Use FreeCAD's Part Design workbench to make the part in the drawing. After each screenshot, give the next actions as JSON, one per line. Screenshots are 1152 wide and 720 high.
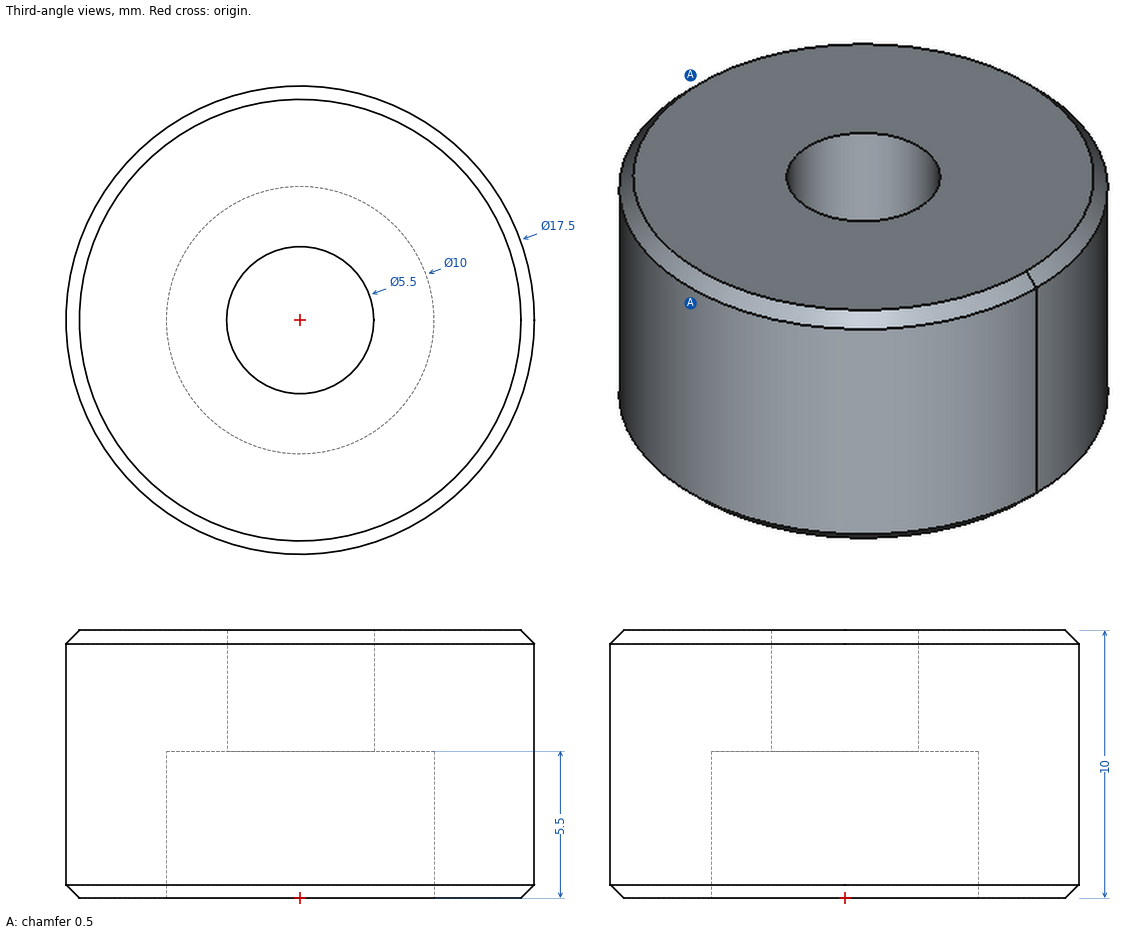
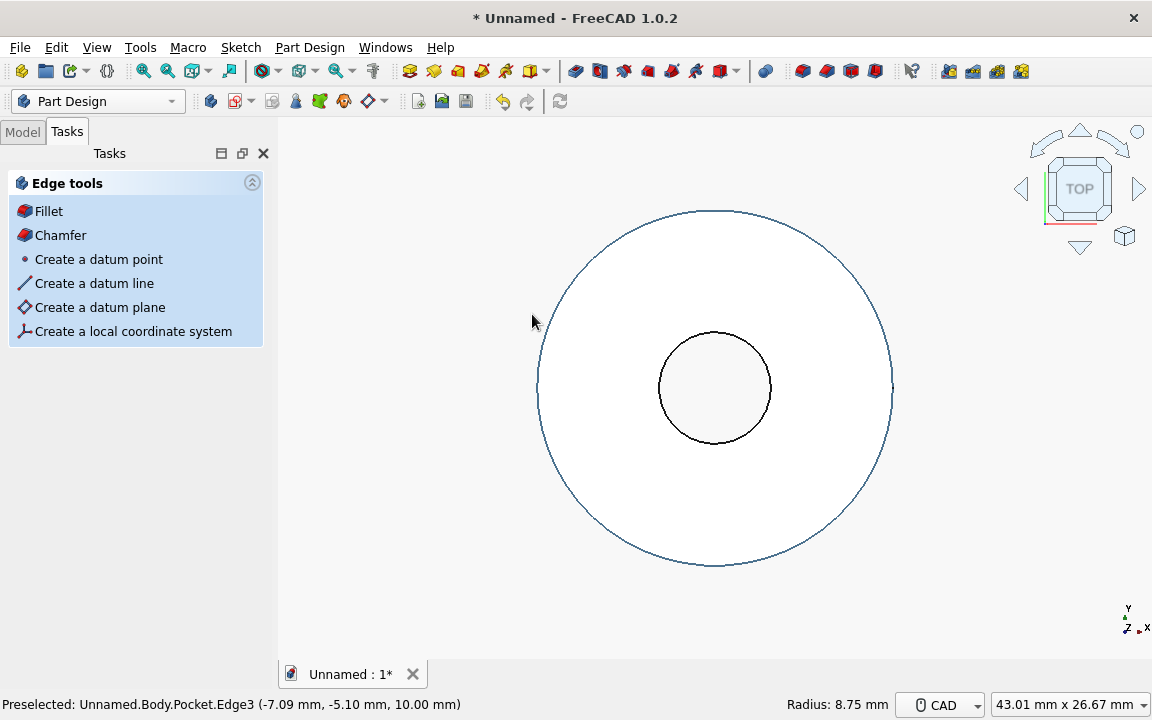
{"action": "key", "text": "1"}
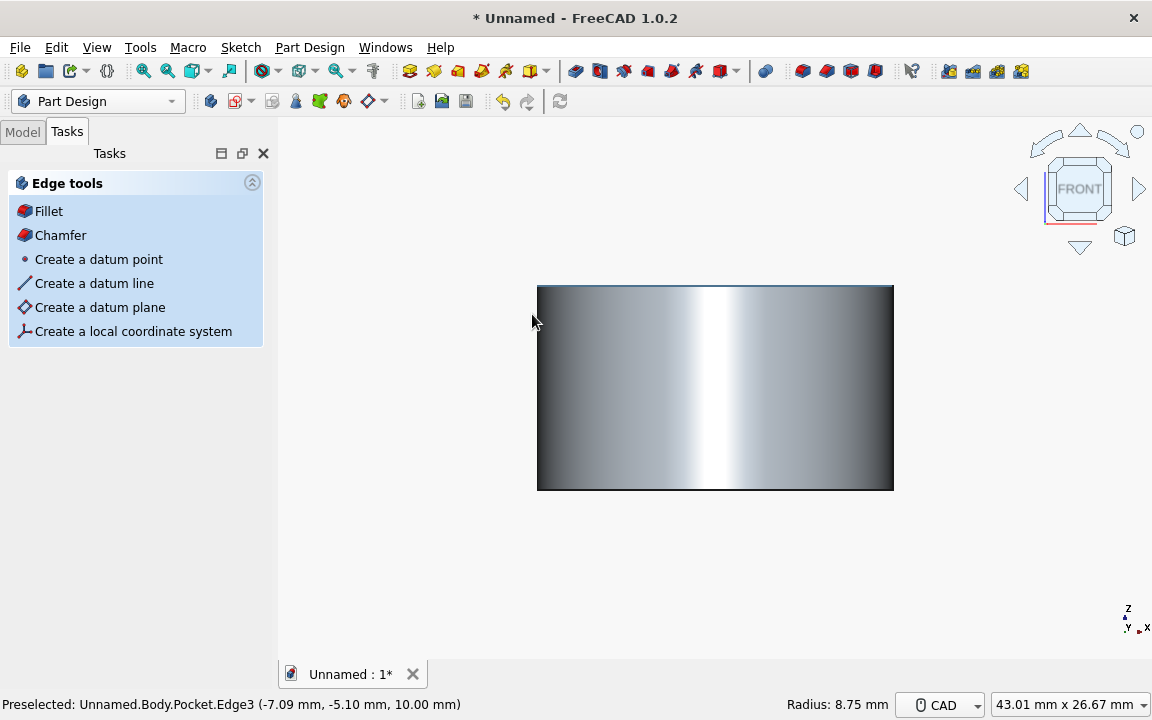
{"action": "left_click", "coordinate": [144, 72]}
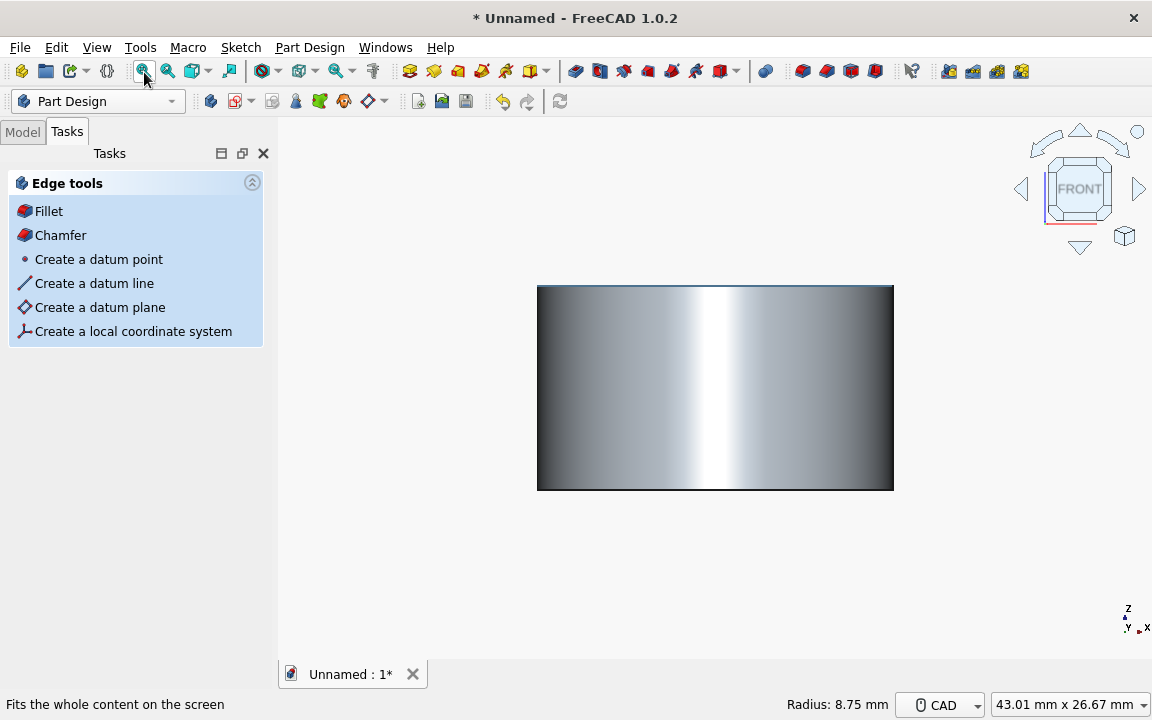
{"action": "left_click", "coordinate": [571, 489], "text": "ctrl"}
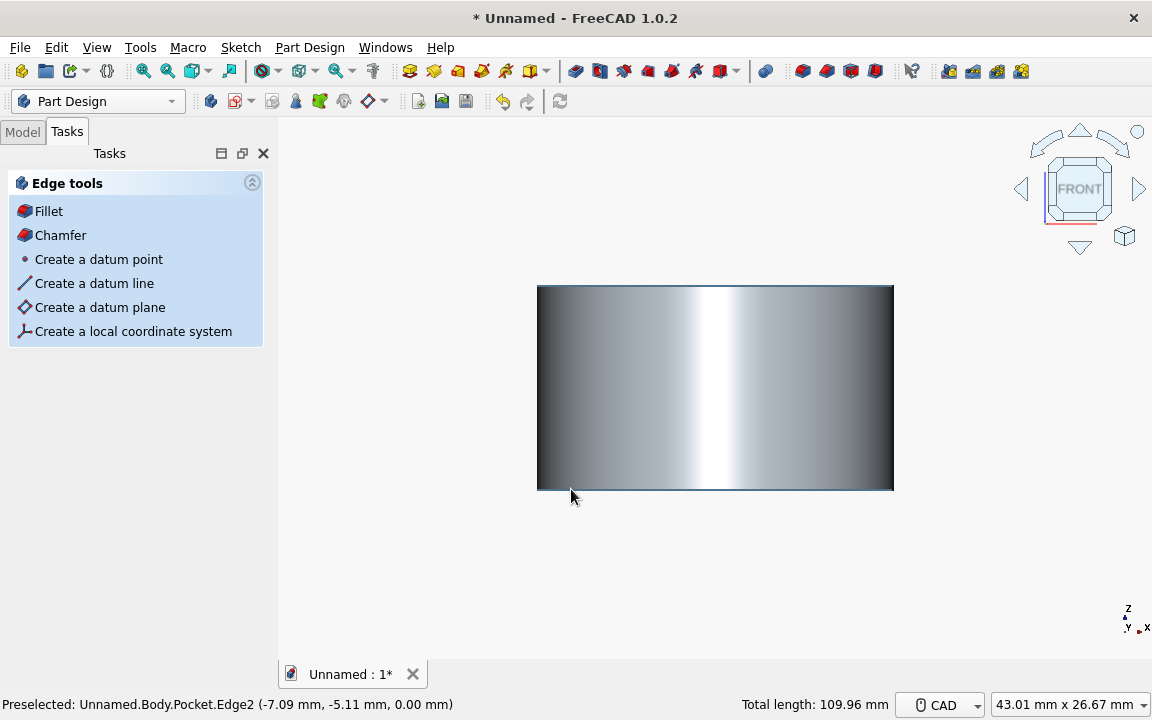
{"action": "left_click", "coordinate": [828, 72]}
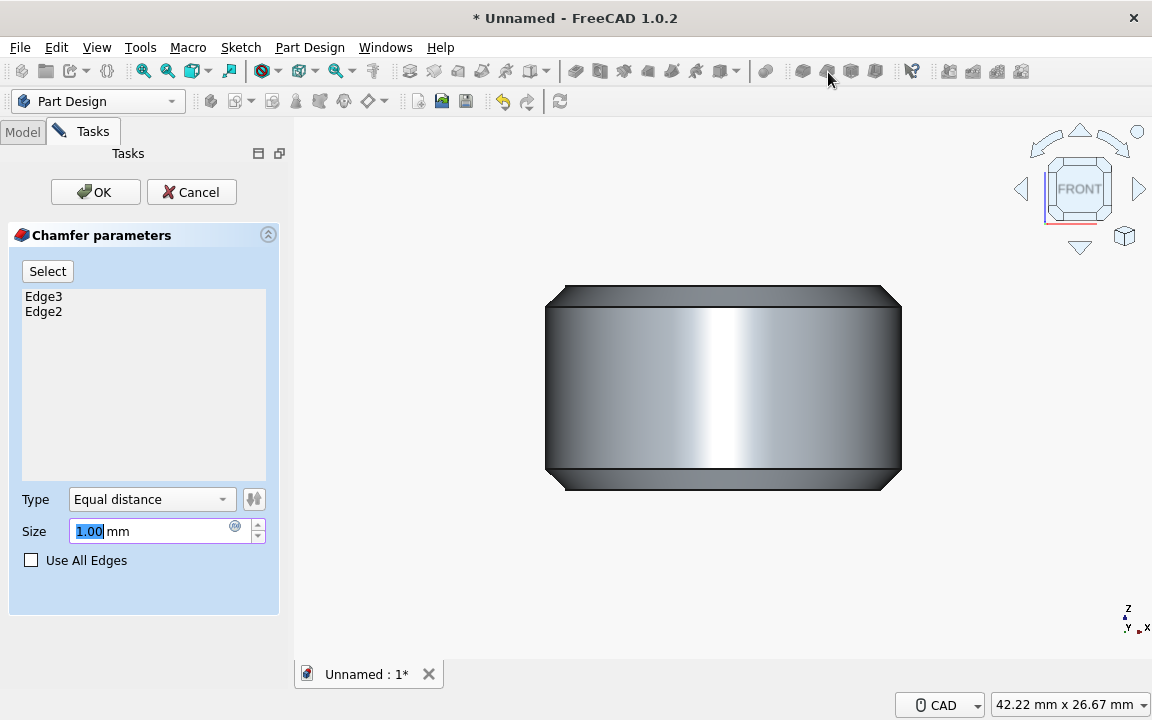
{"action": "type", "text": "0.5"}
{"action": "key", "text": "Tab"}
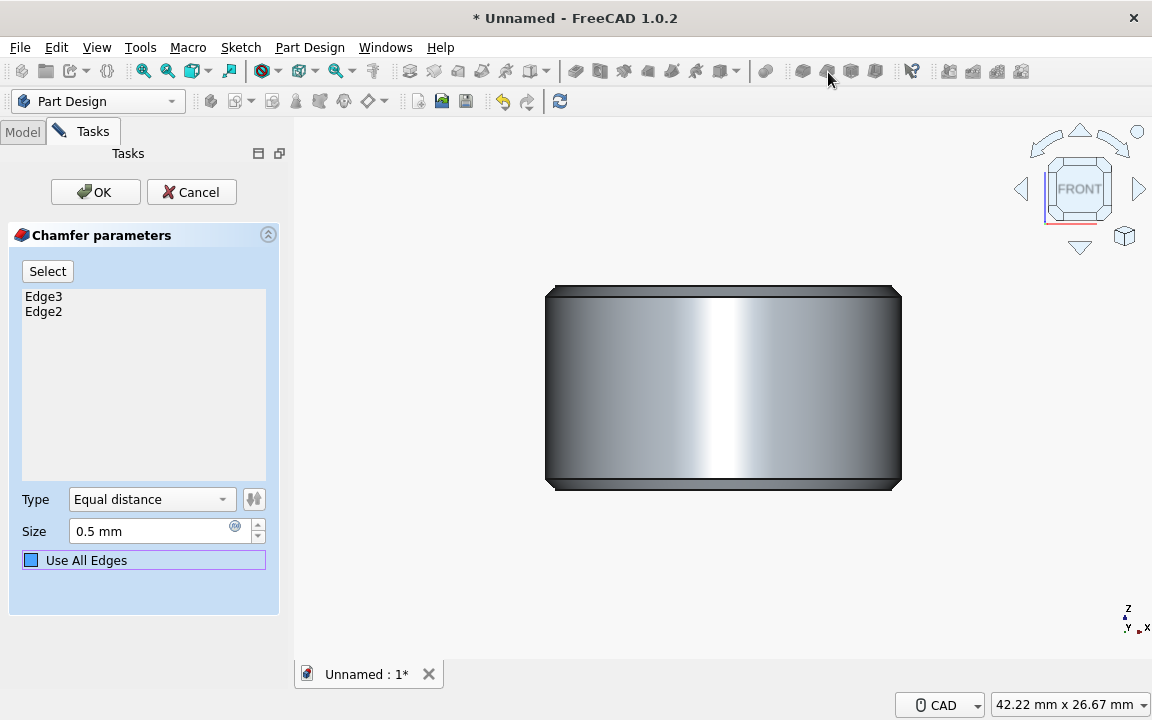
{"action": "left_click", "coordinate": [96, 192]}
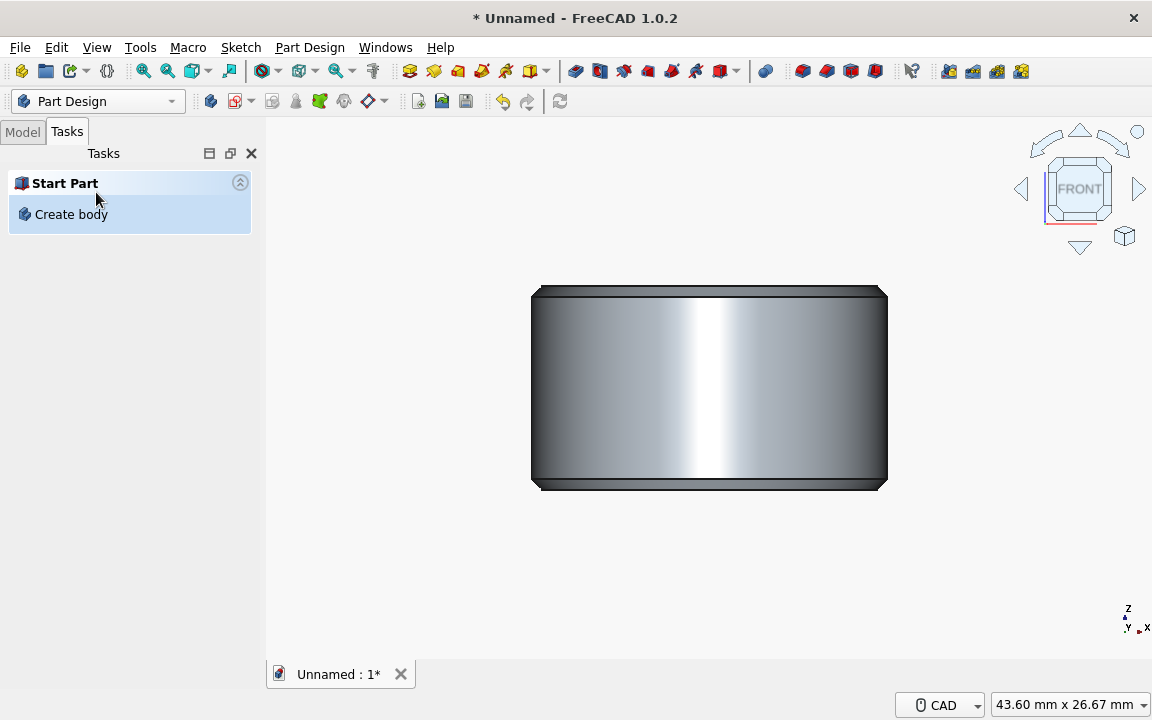
{"action": "key", "text": "0"}